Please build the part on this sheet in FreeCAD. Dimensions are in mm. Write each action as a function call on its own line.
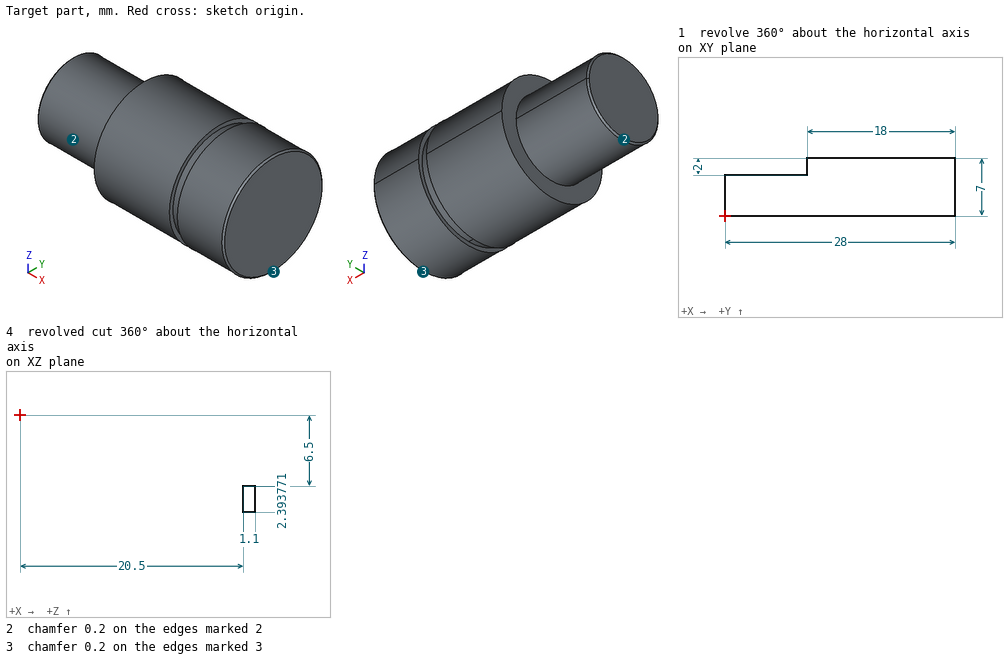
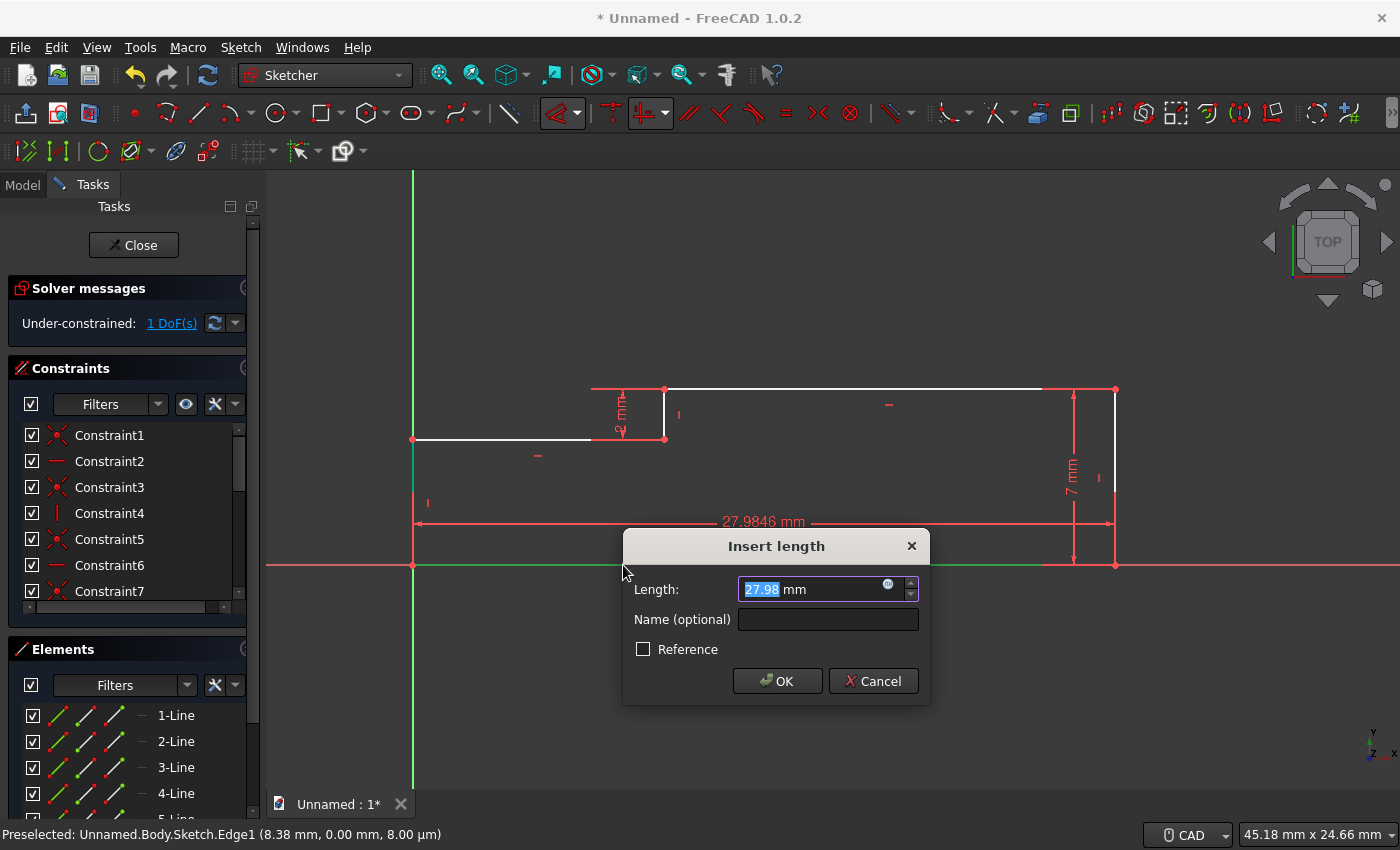
text(28)
key(Return)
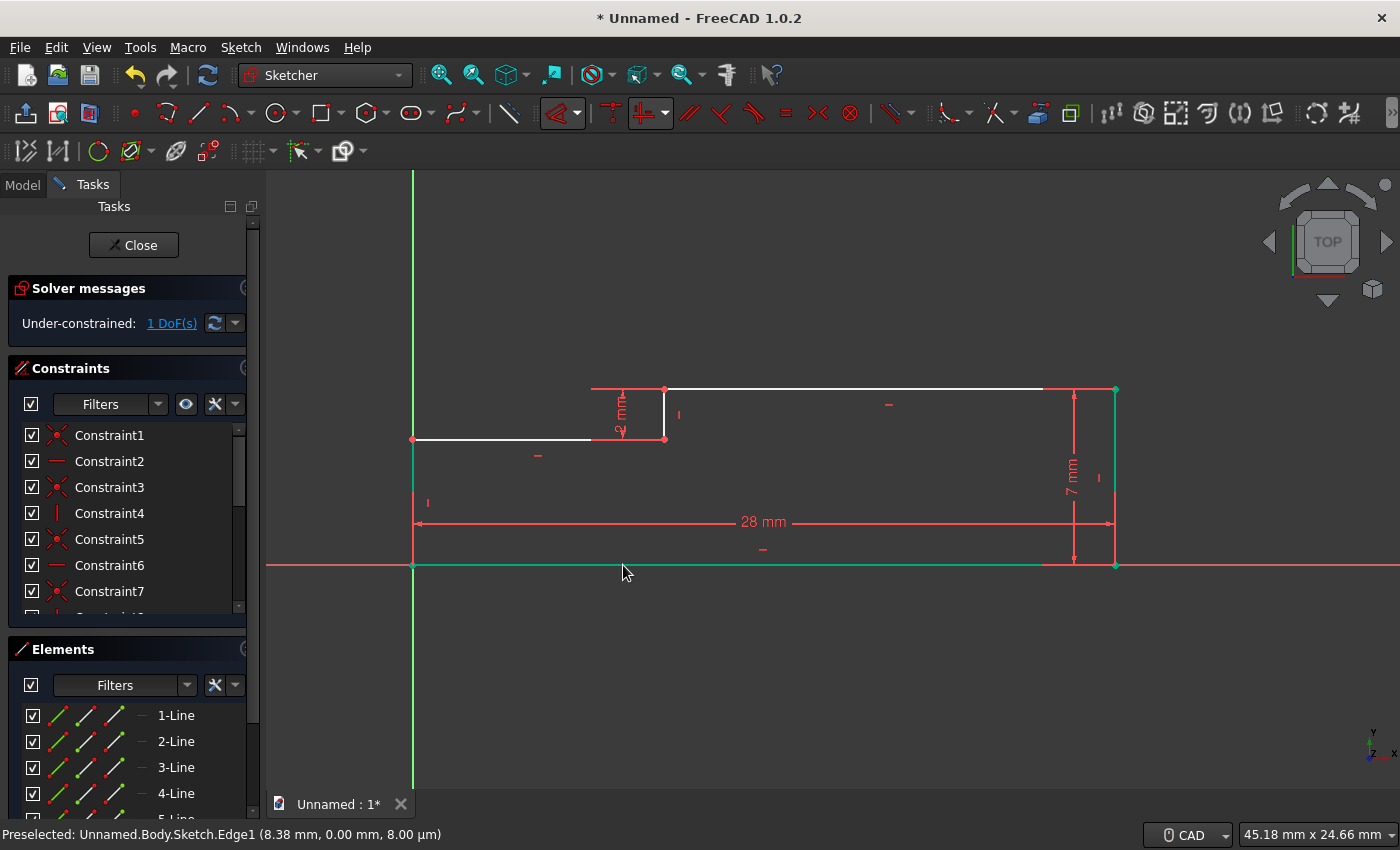
click(980, 389)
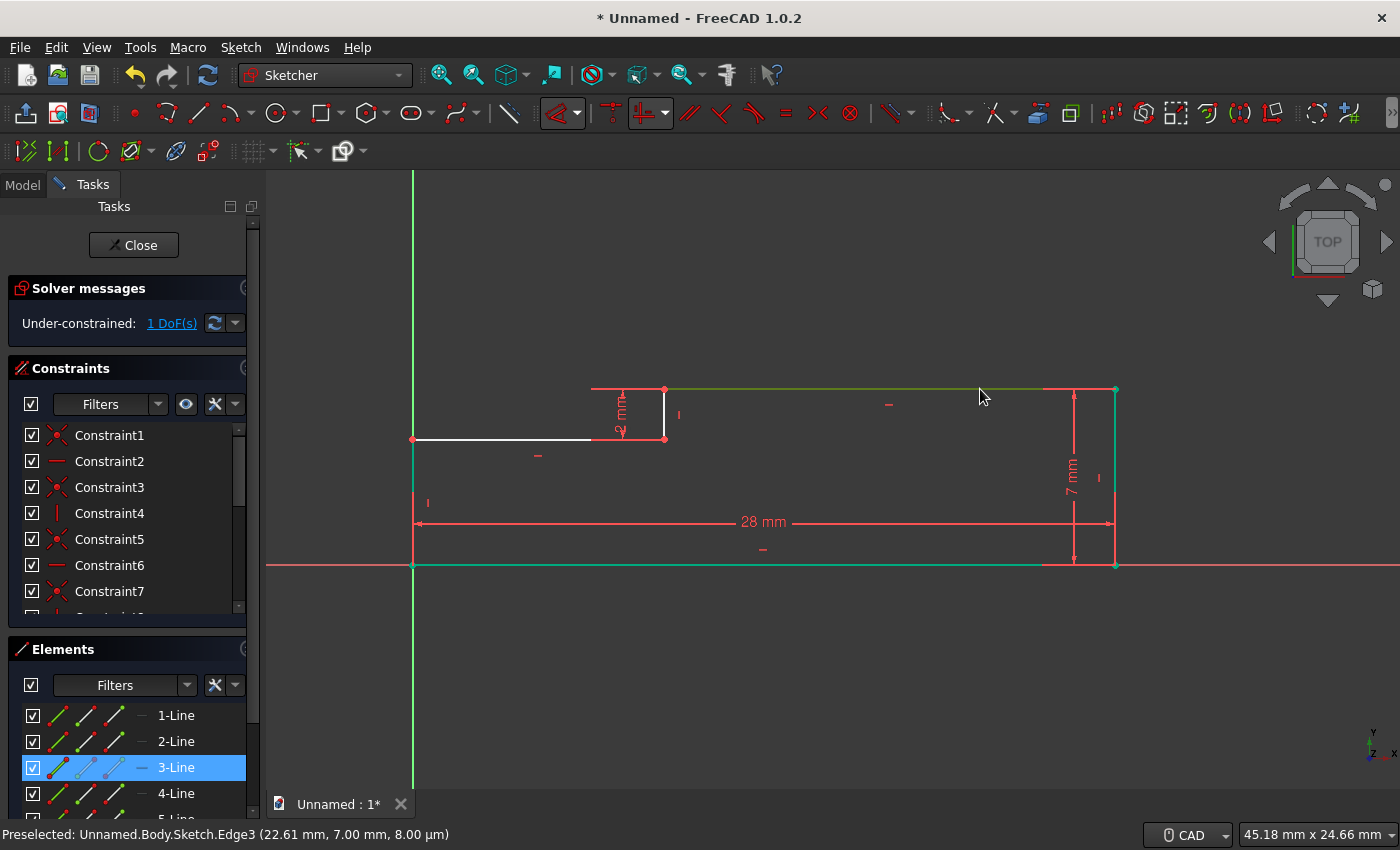
key(l)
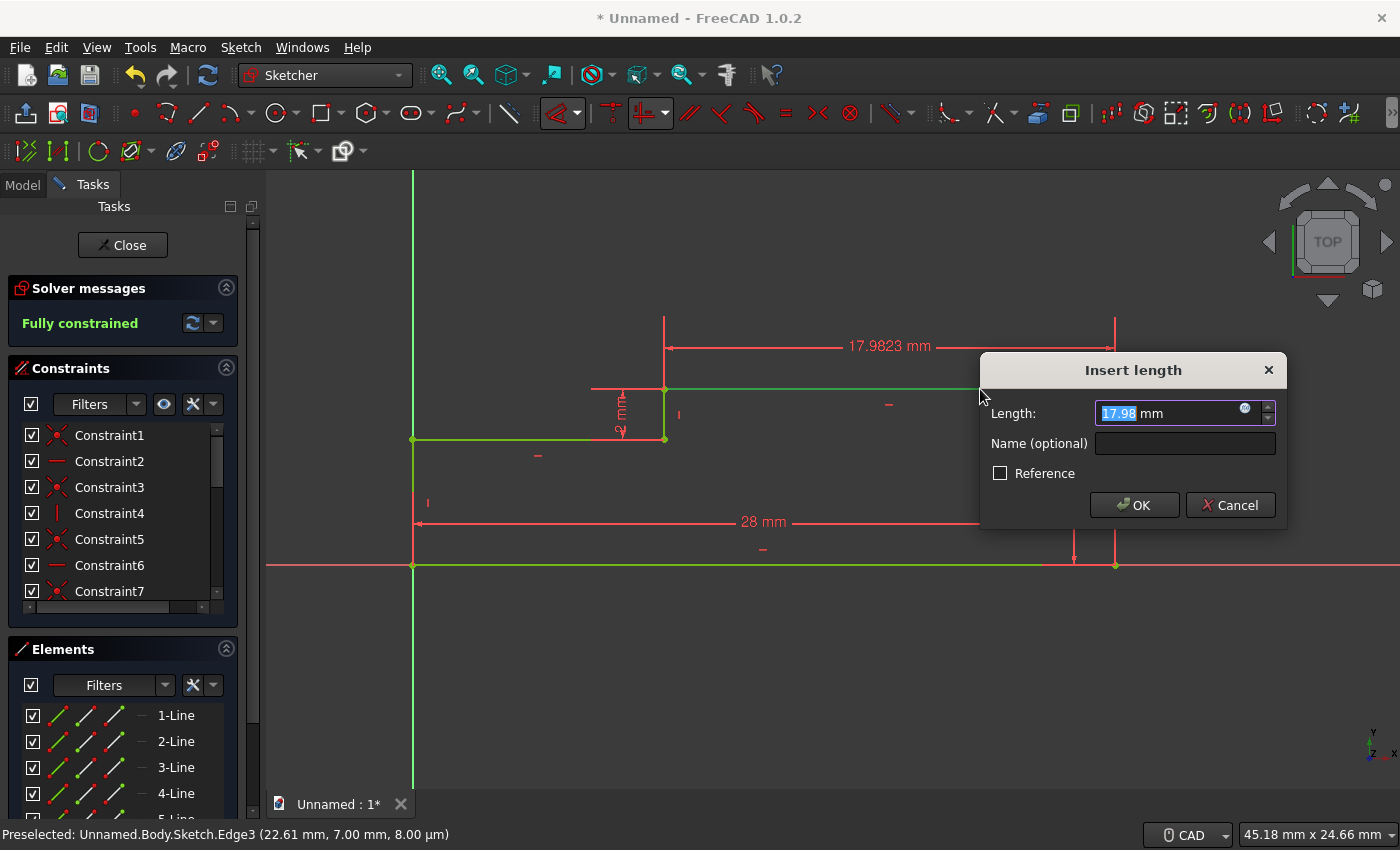
text(18)
key(Return)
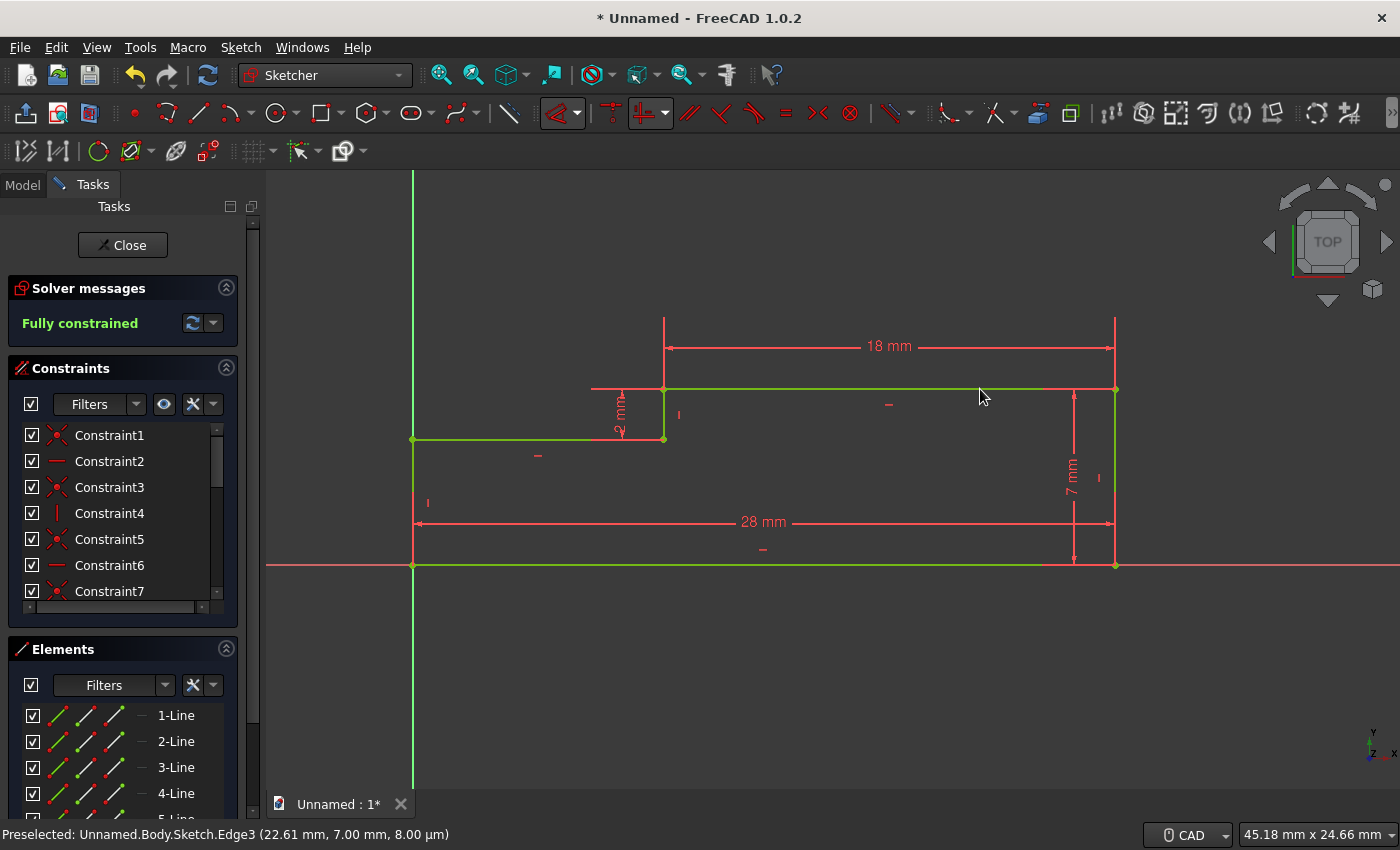
click(123, 245)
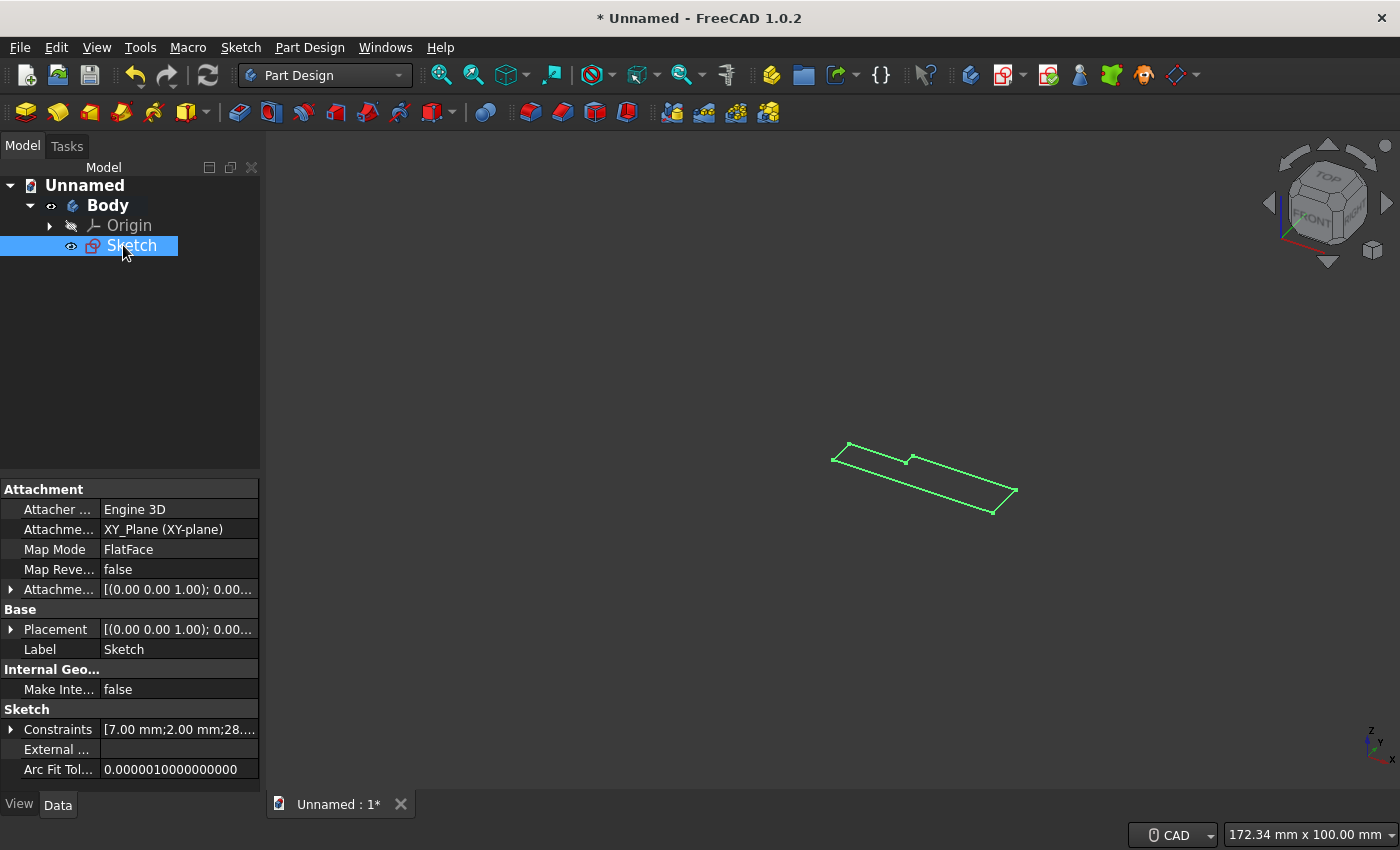
click(58, 112)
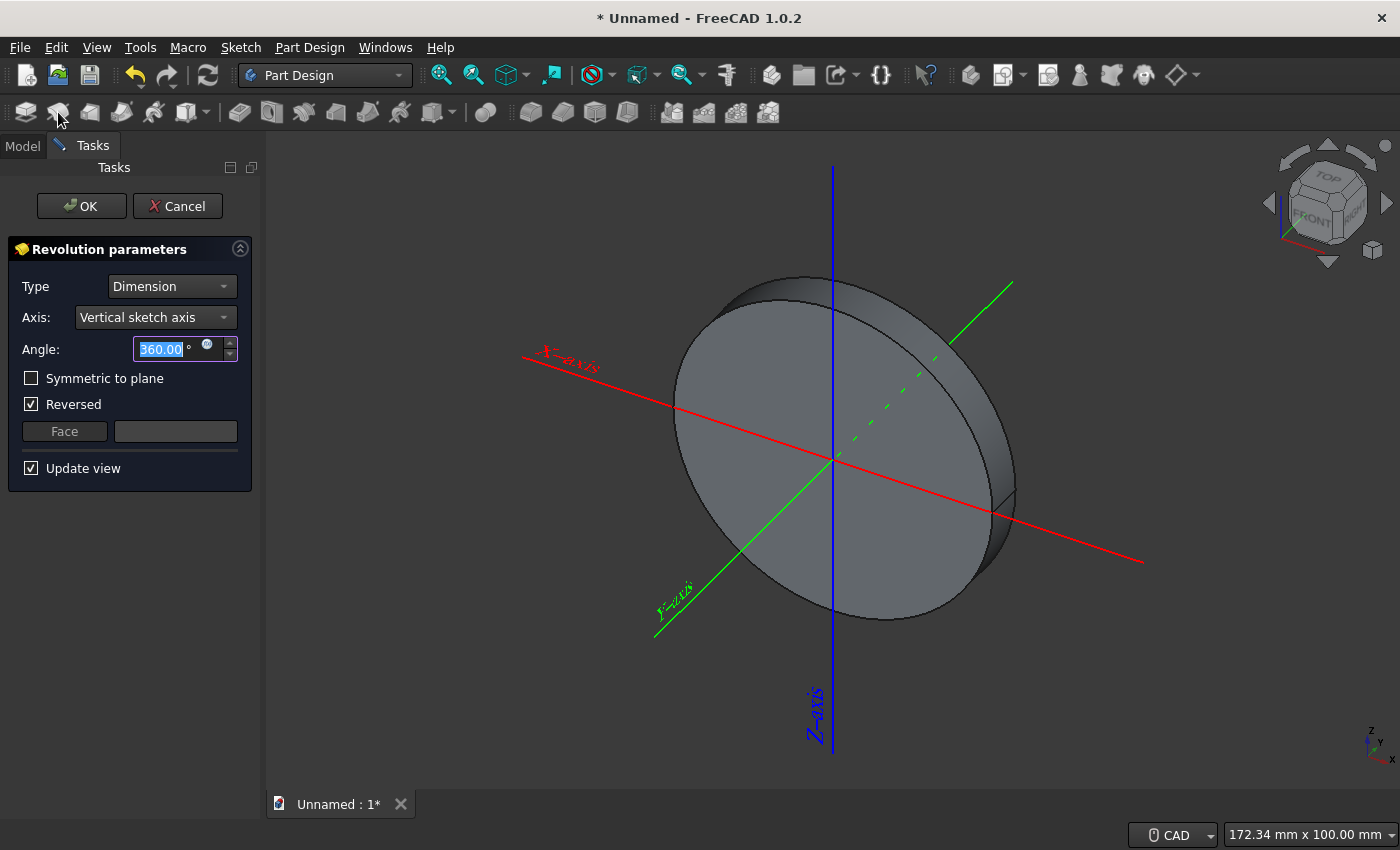
click(156, 318)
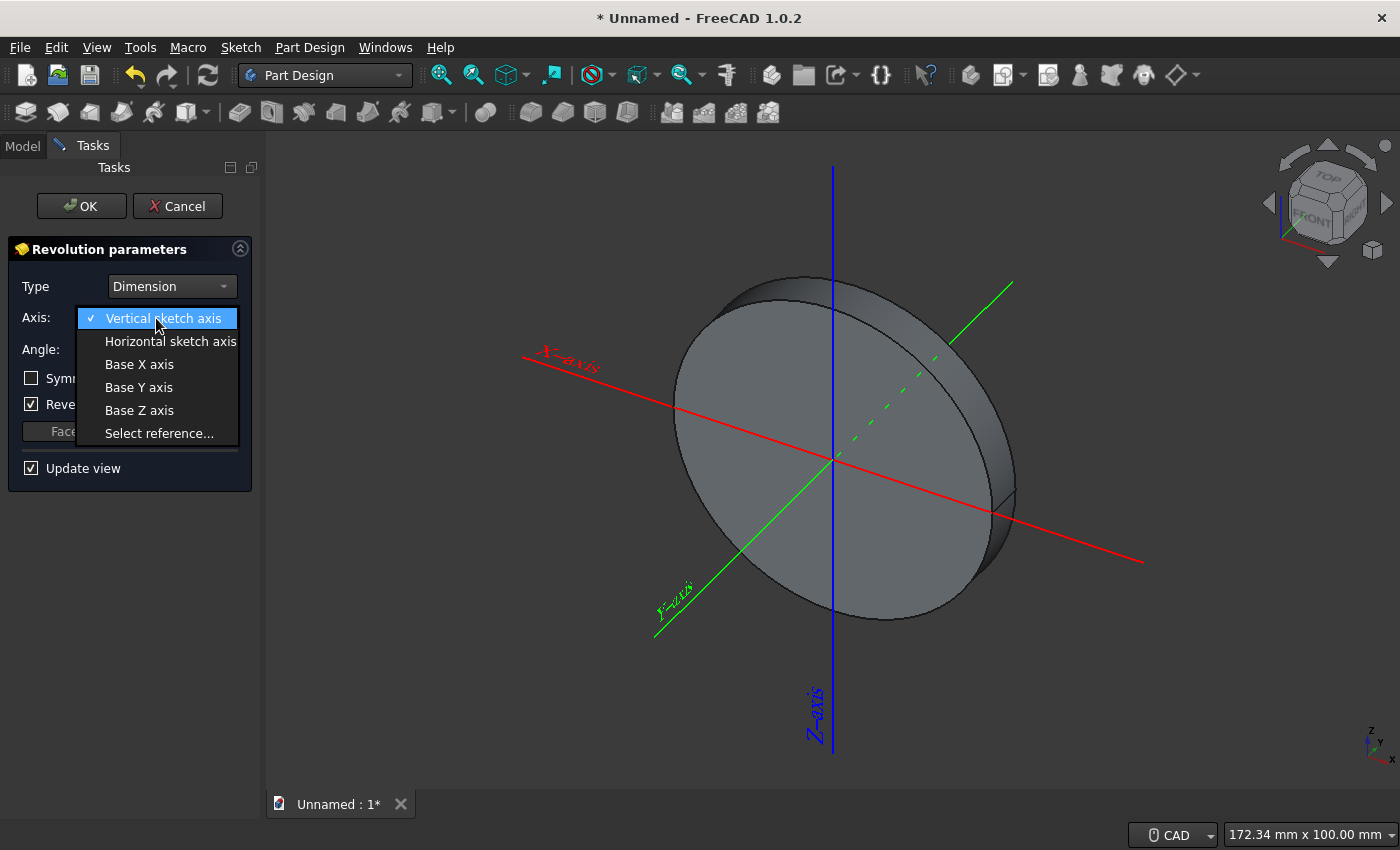
click(156, 342)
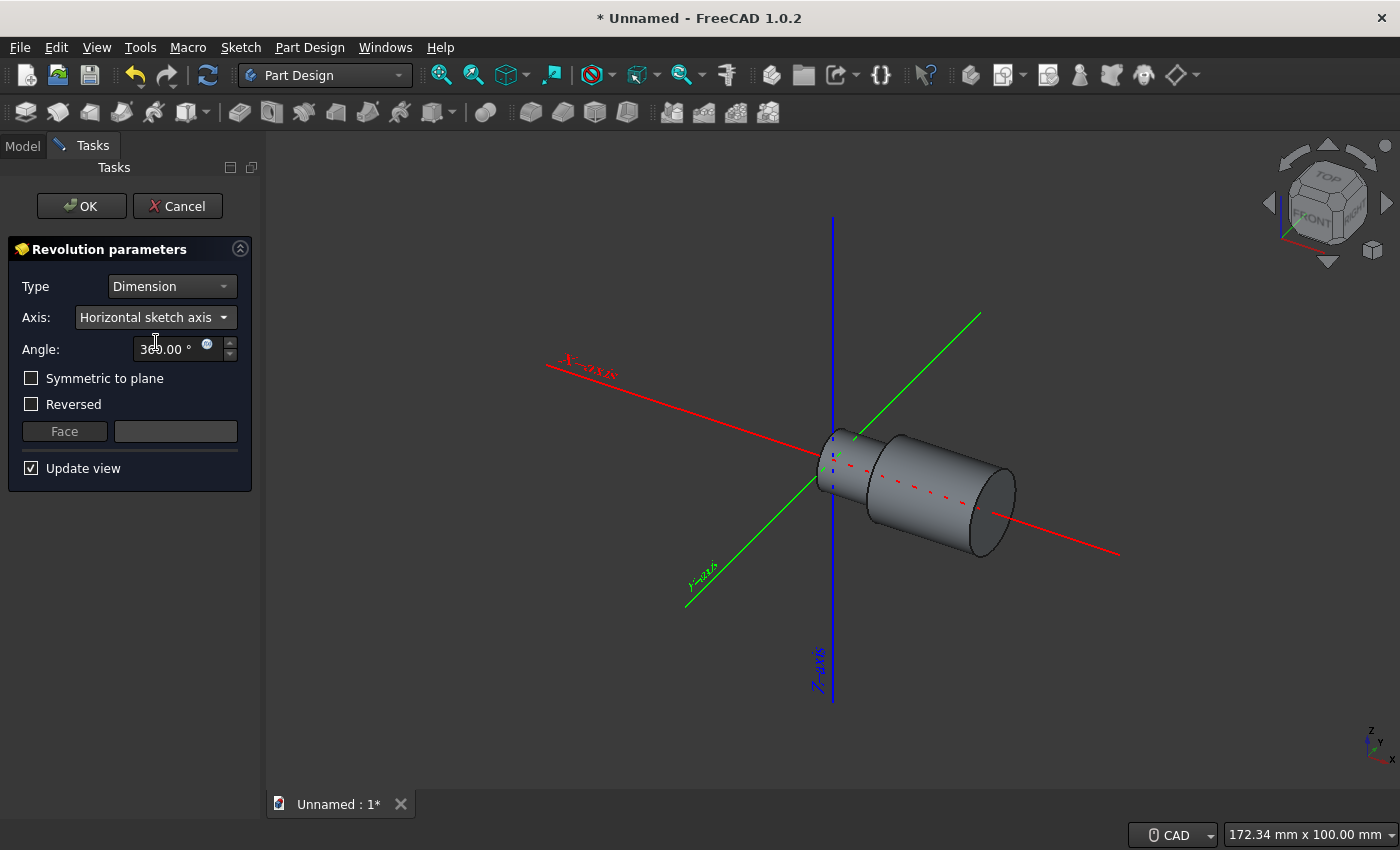
click(82, 206)